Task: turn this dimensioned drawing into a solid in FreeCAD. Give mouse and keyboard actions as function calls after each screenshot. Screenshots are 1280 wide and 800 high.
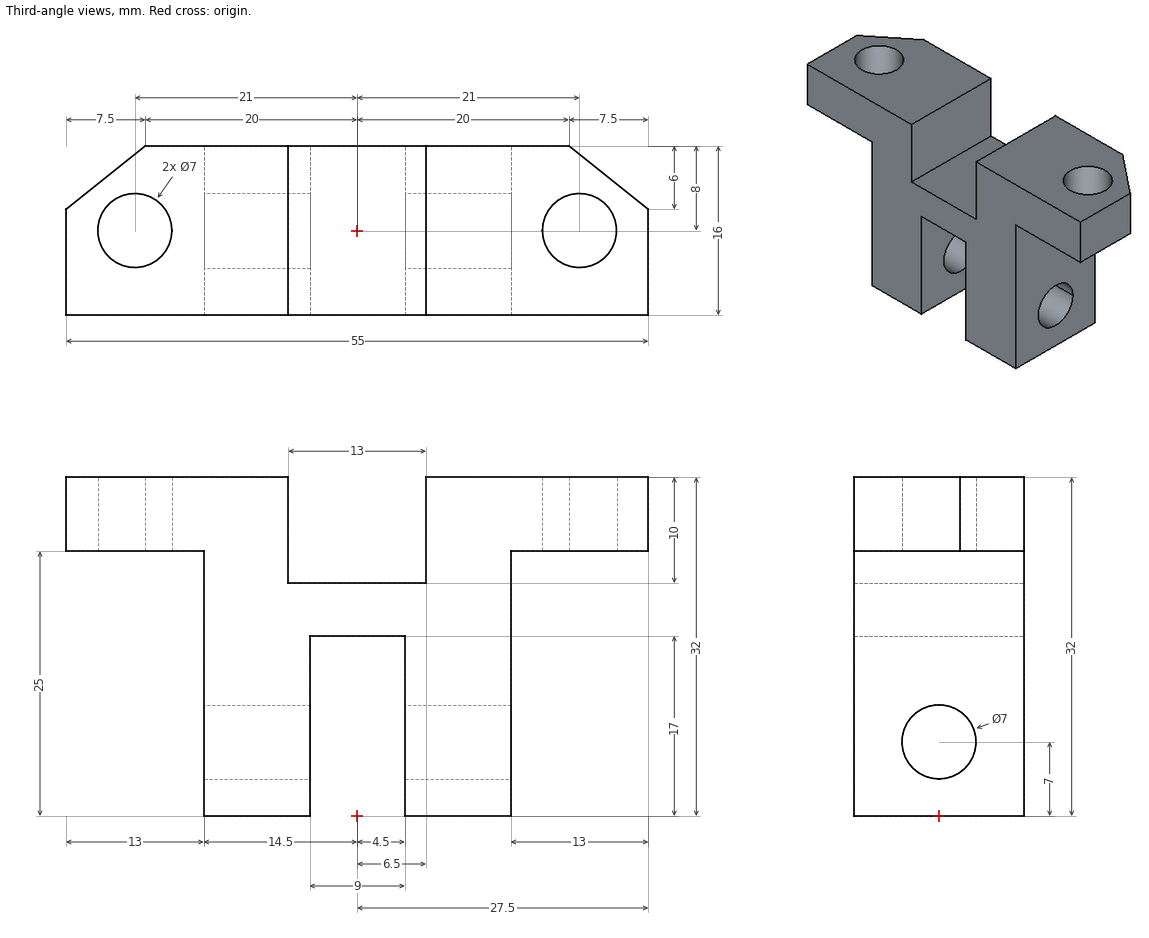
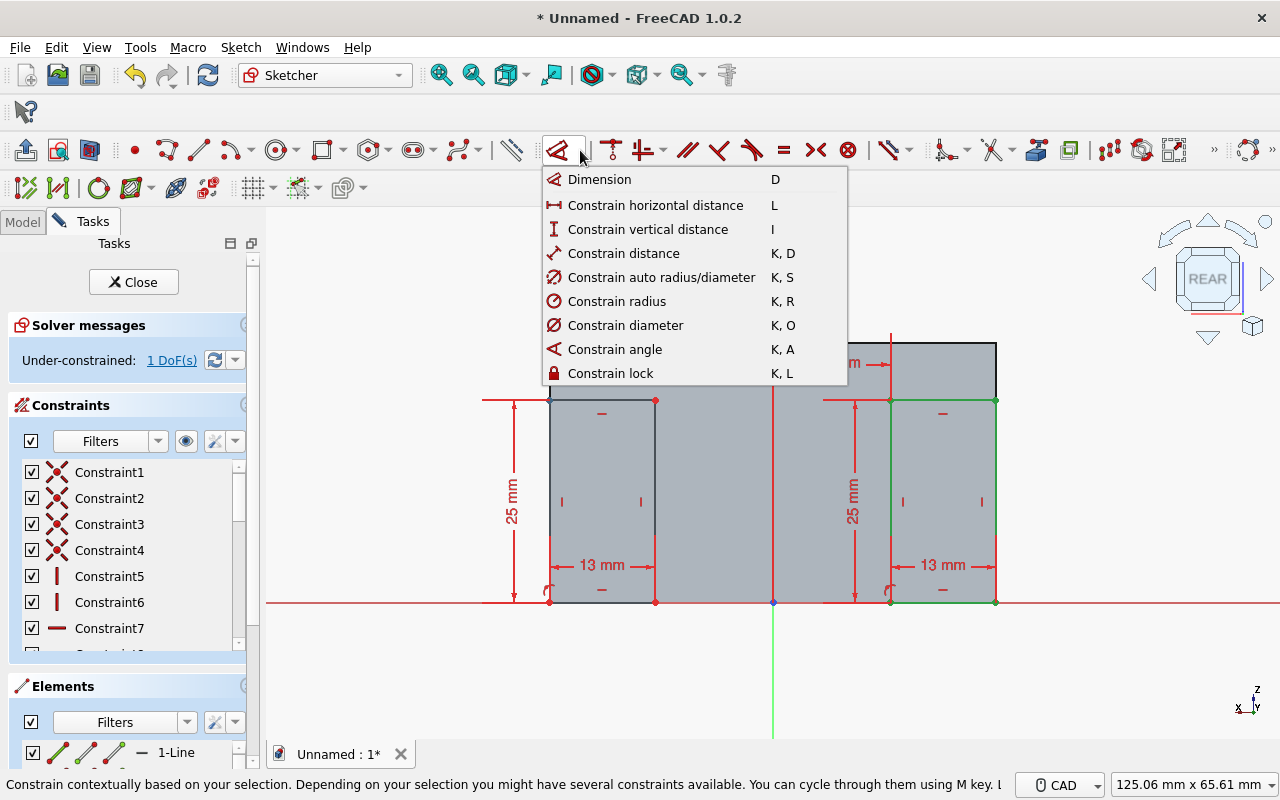
click(695, 205)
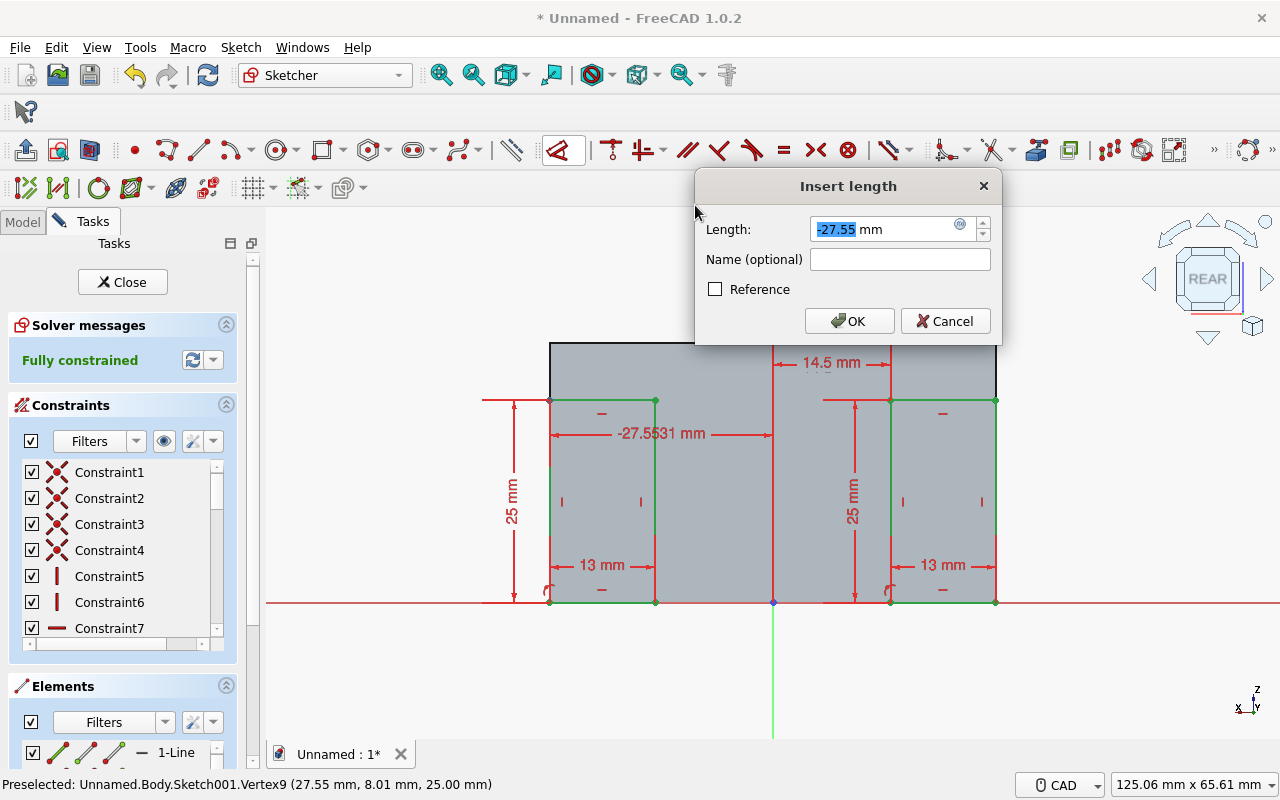
text(-27.5)
key(Return)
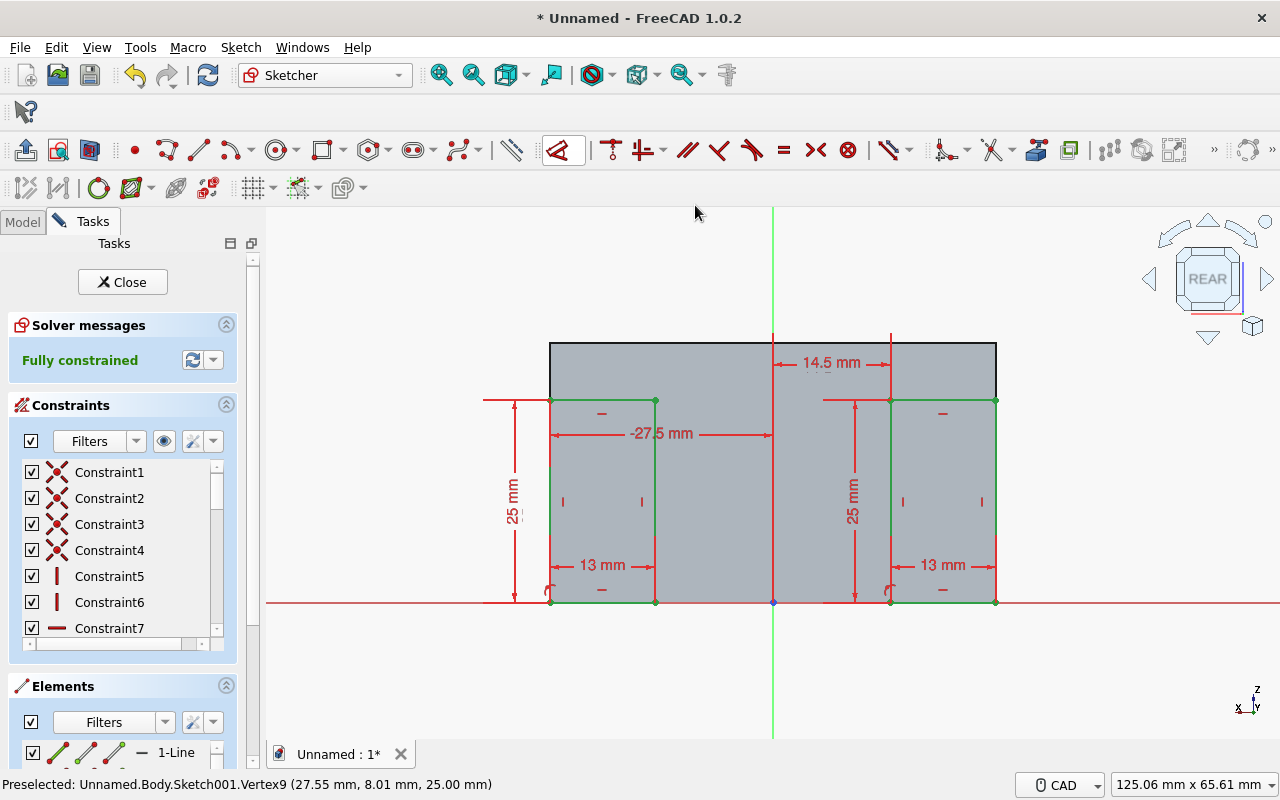
click(123, 282)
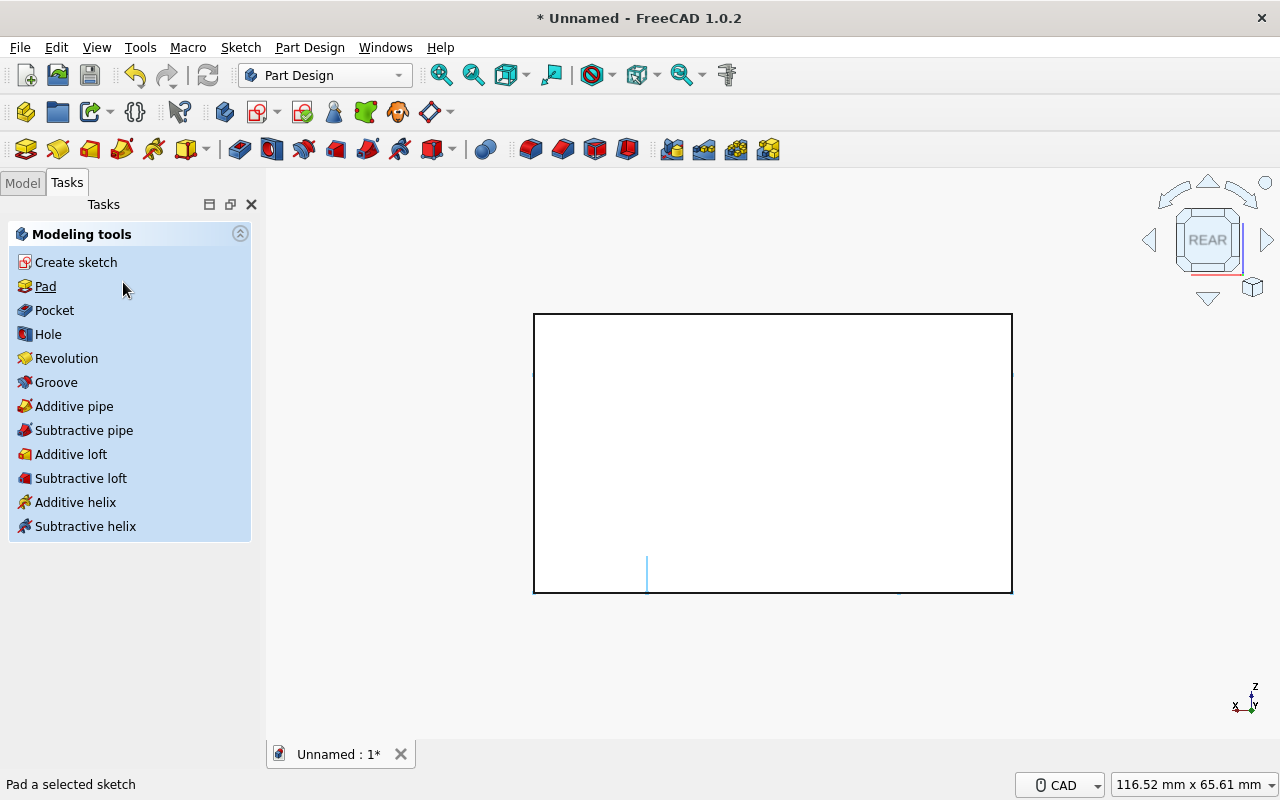
click(240, 150)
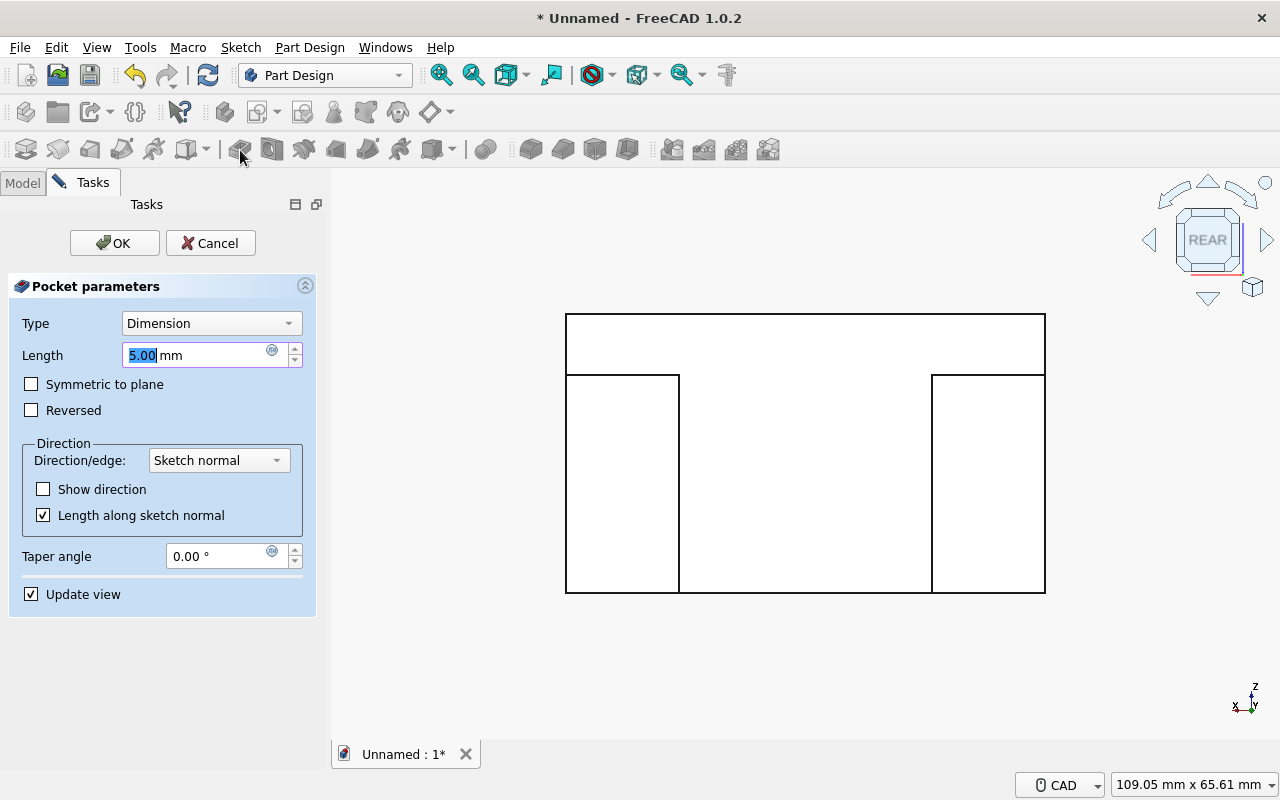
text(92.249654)
key(Tab)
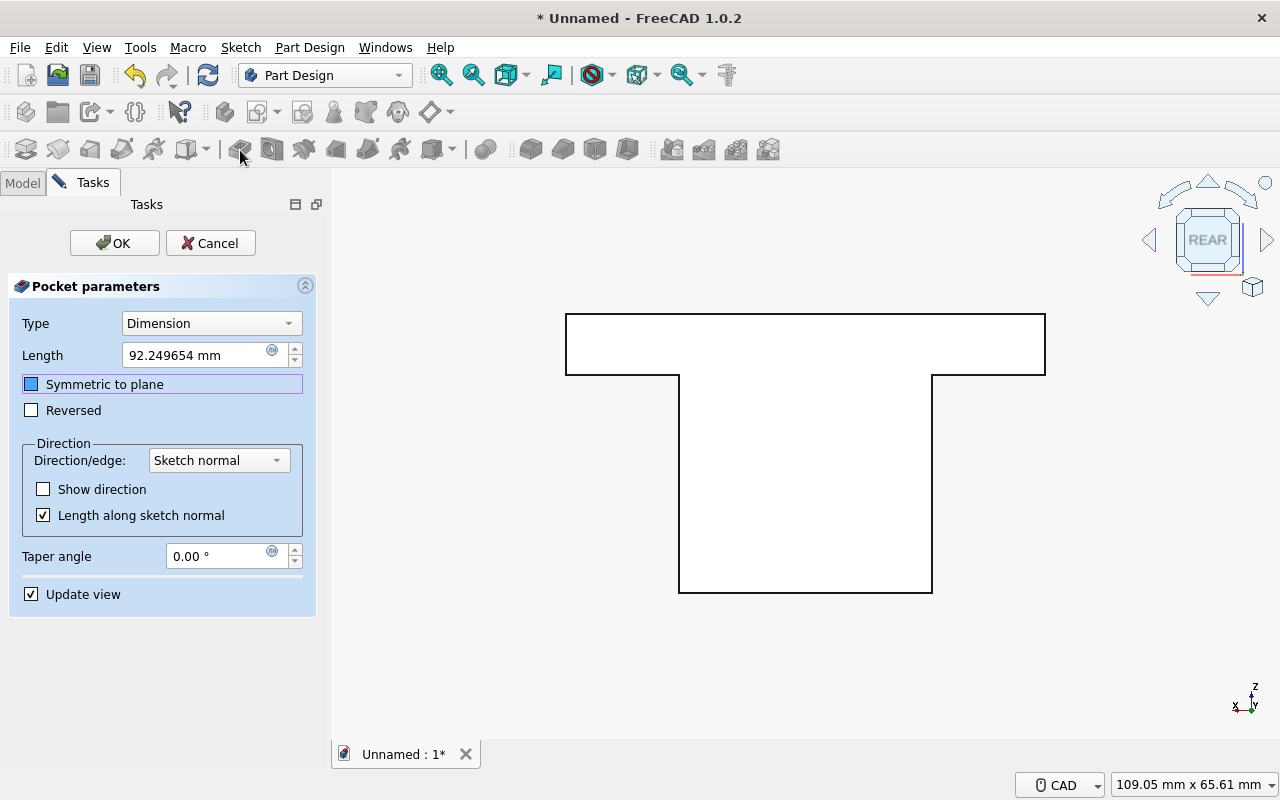
click(30, 384)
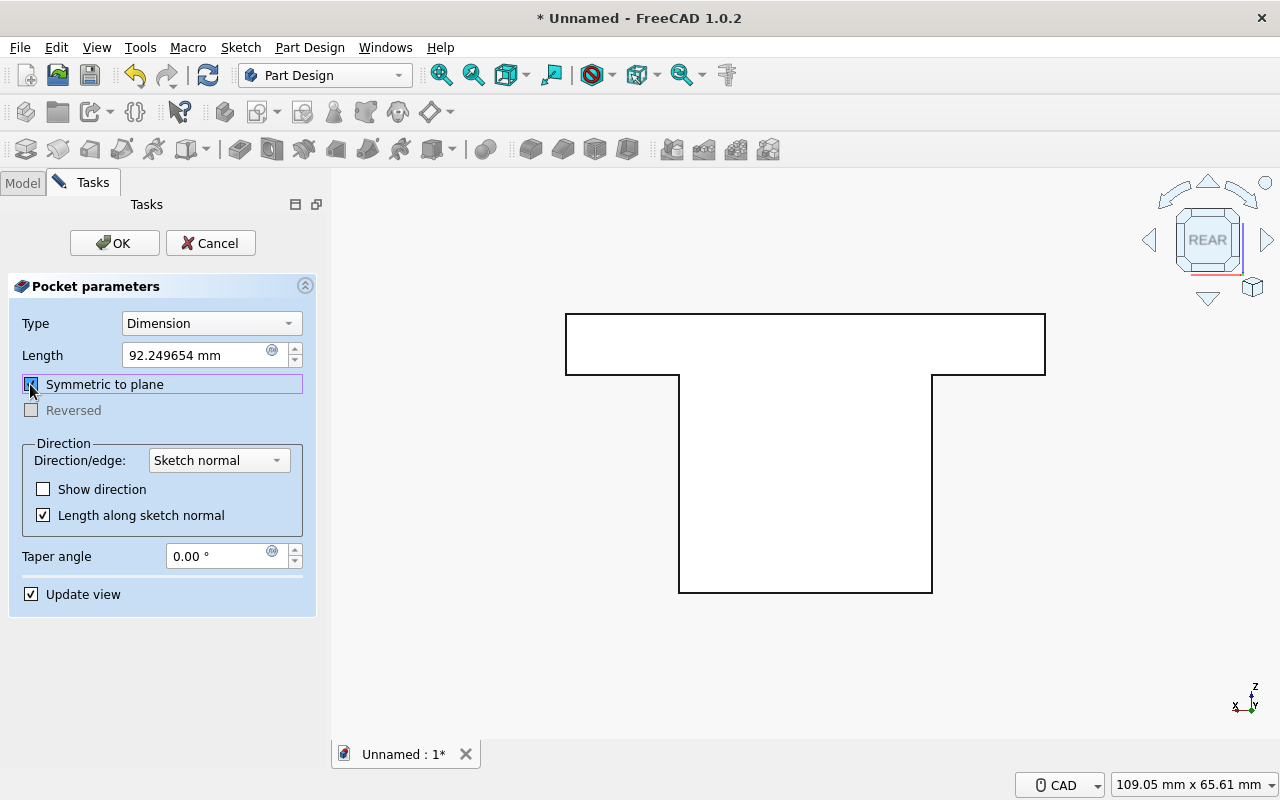
click(115, 243)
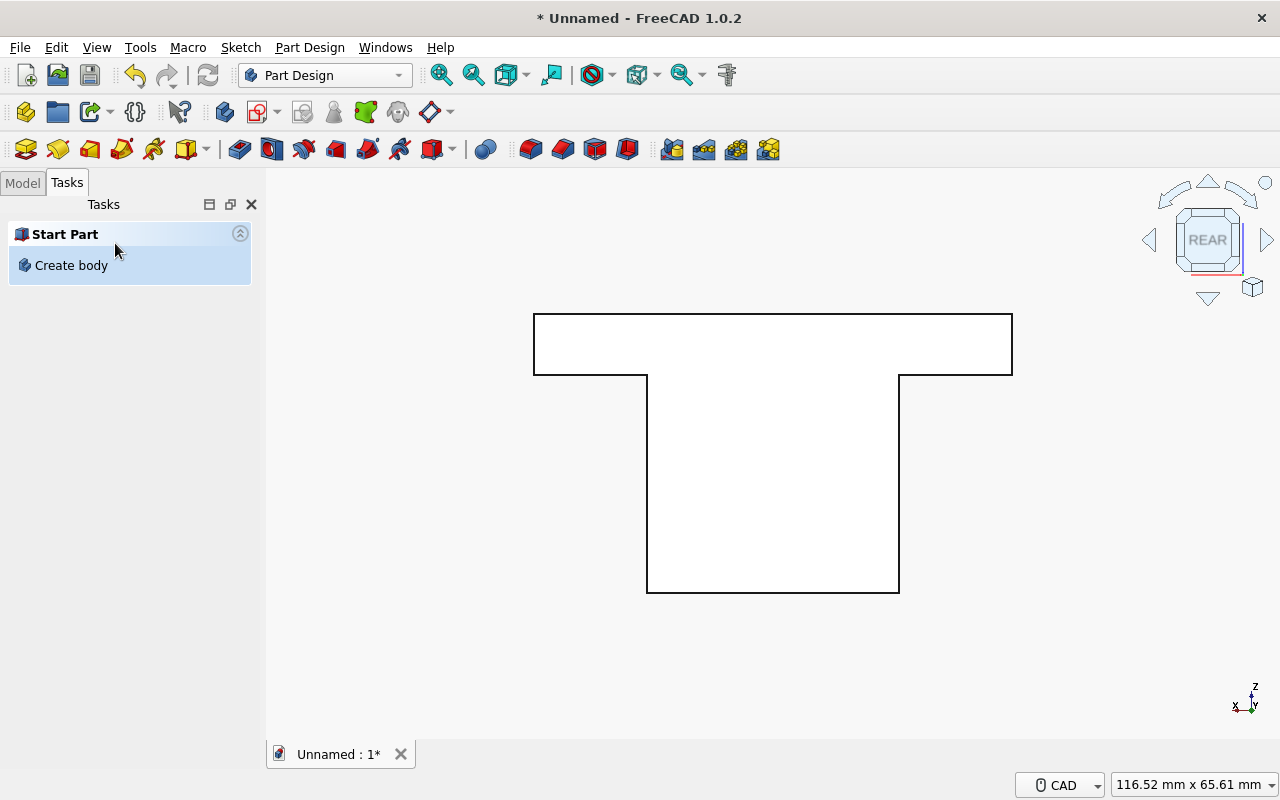
click(773, 453)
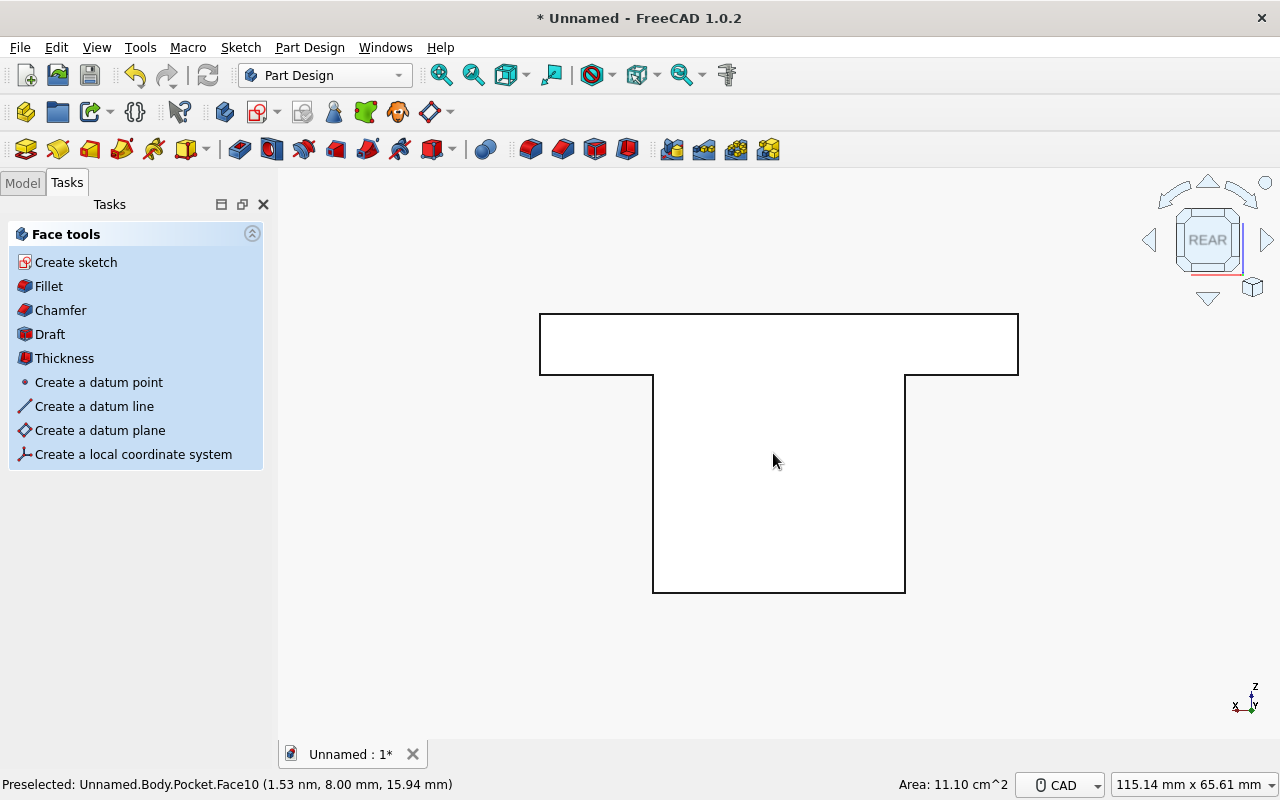
click(258, 112)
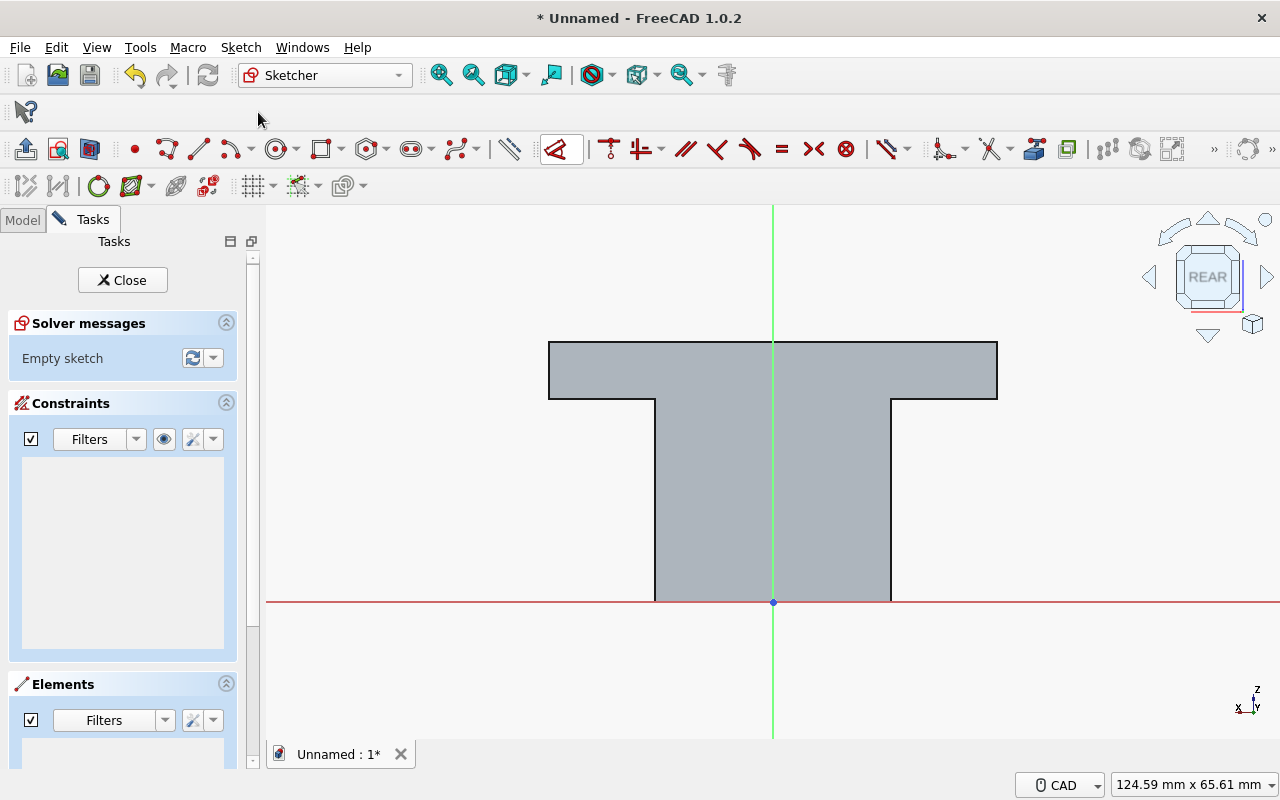
click(322, 150)